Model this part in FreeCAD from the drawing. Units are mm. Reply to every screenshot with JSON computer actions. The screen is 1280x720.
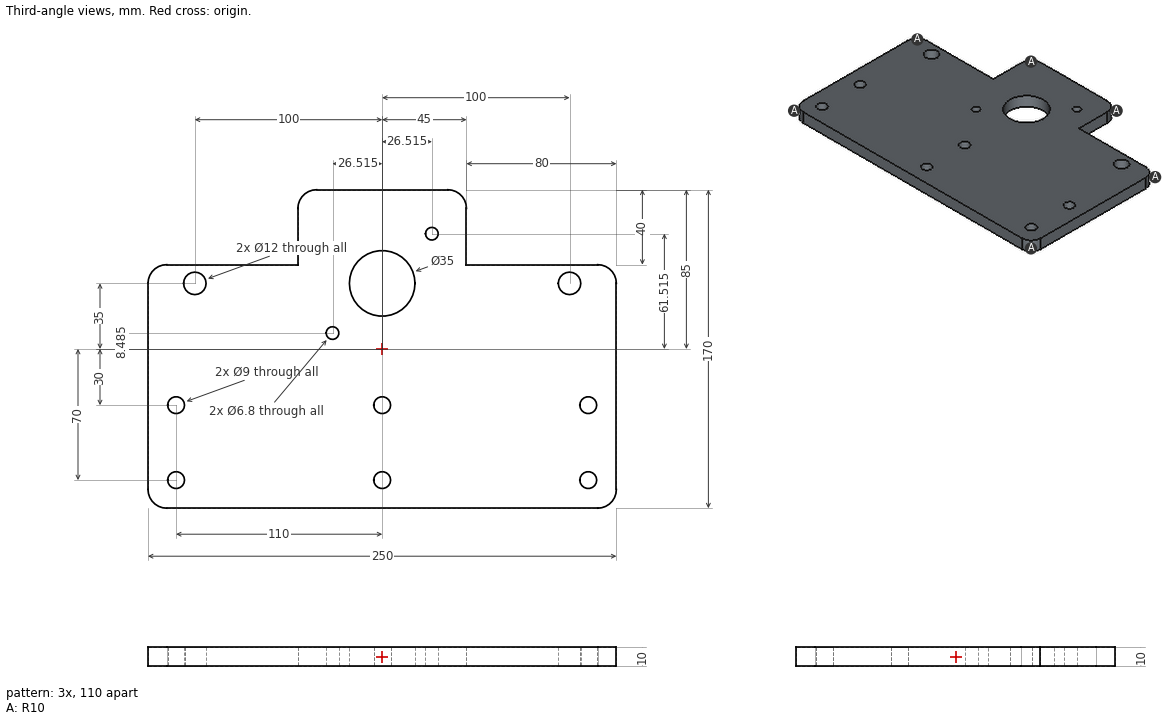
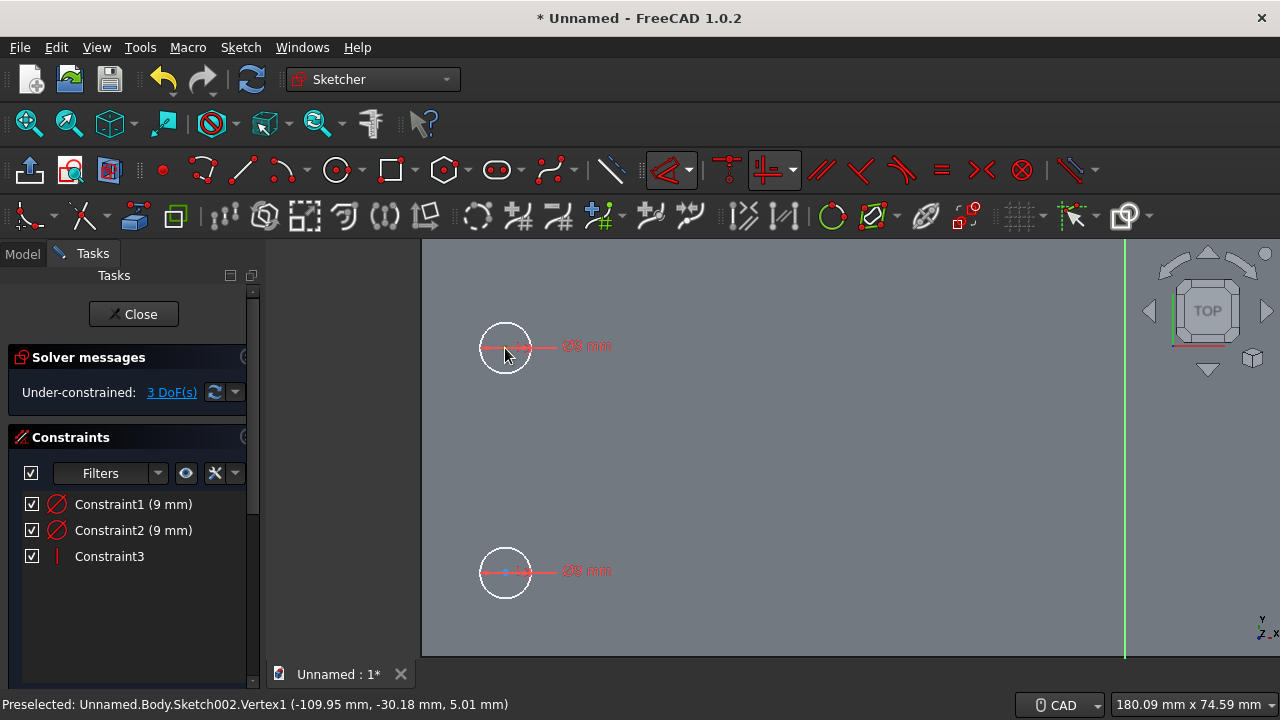
{"action": "left_click", "coordinate": [692, 170]}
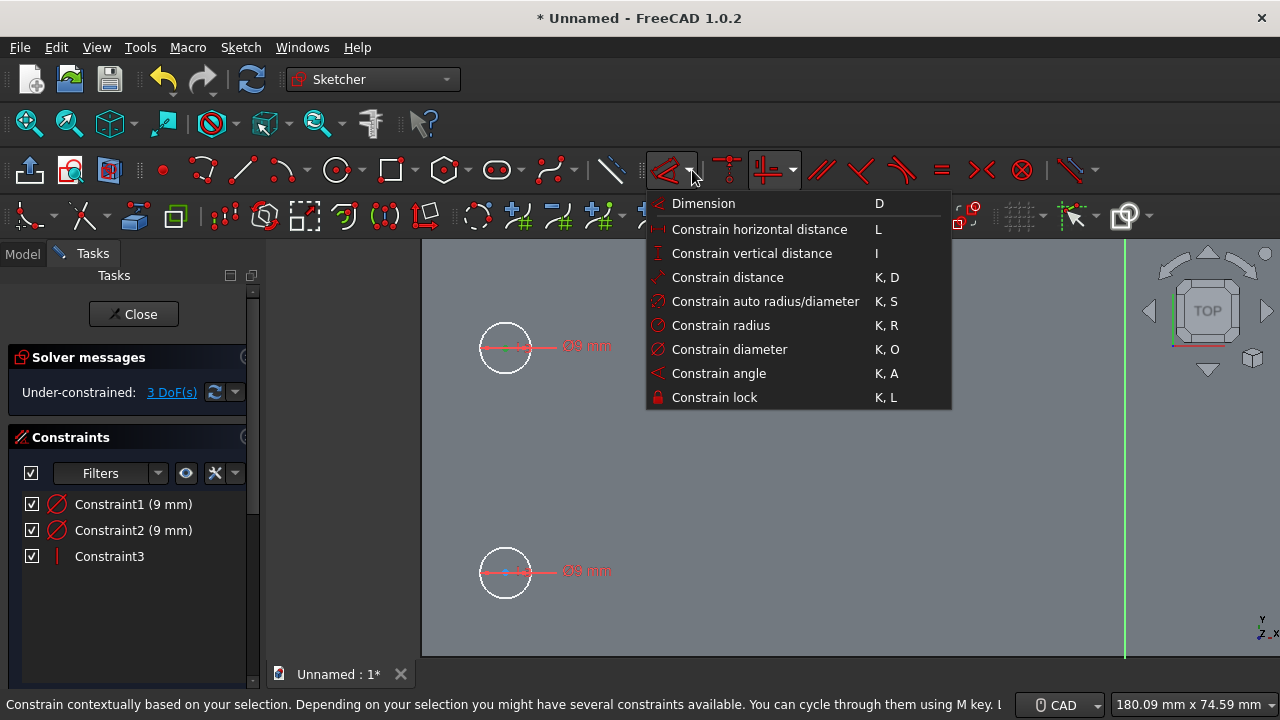
{"action": "left_click", "coordinate": [799, 253]}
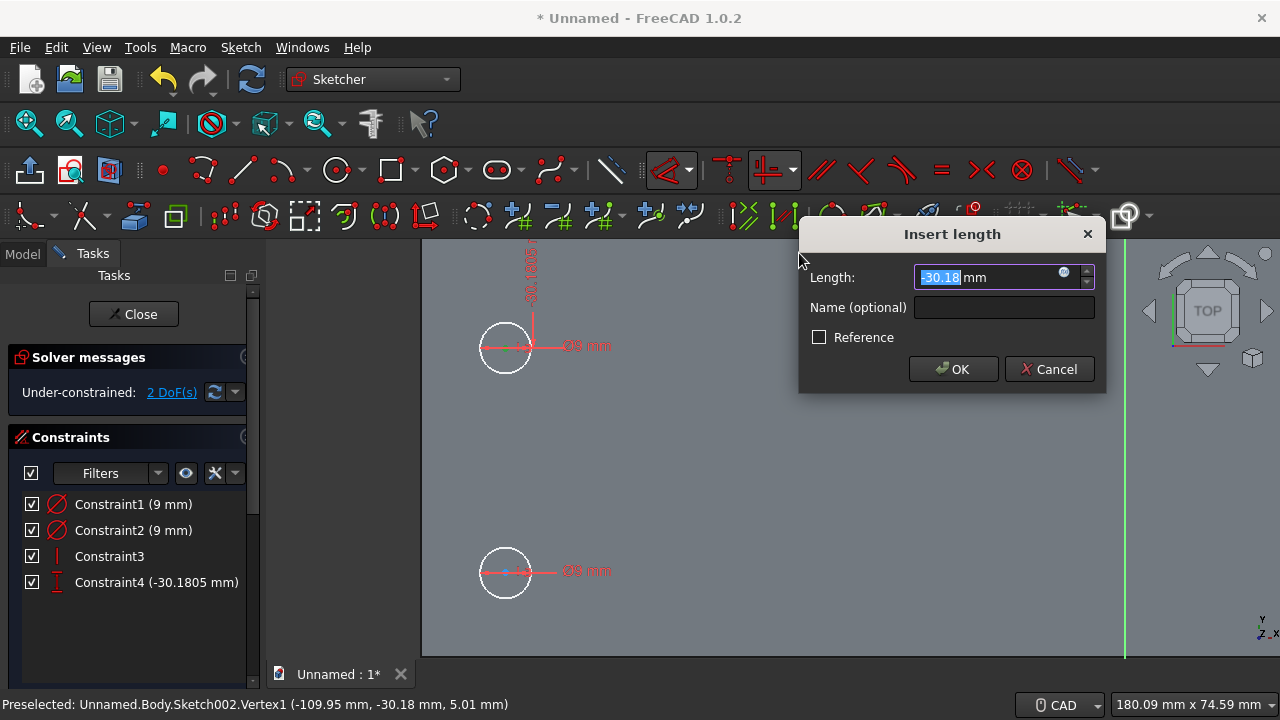
{"action": "type", "text": "-30"}
{"action": "key", "text": "Return"}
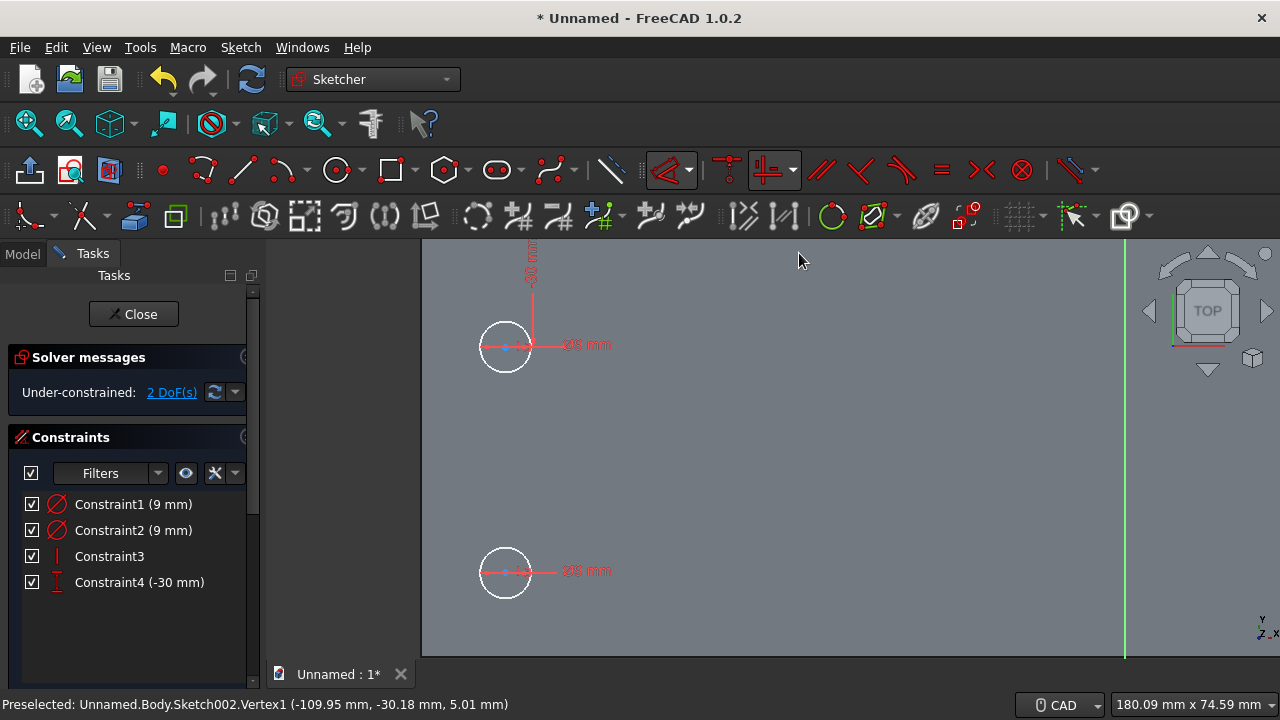
{"action": "left_click", "coordinate": [505, 573]}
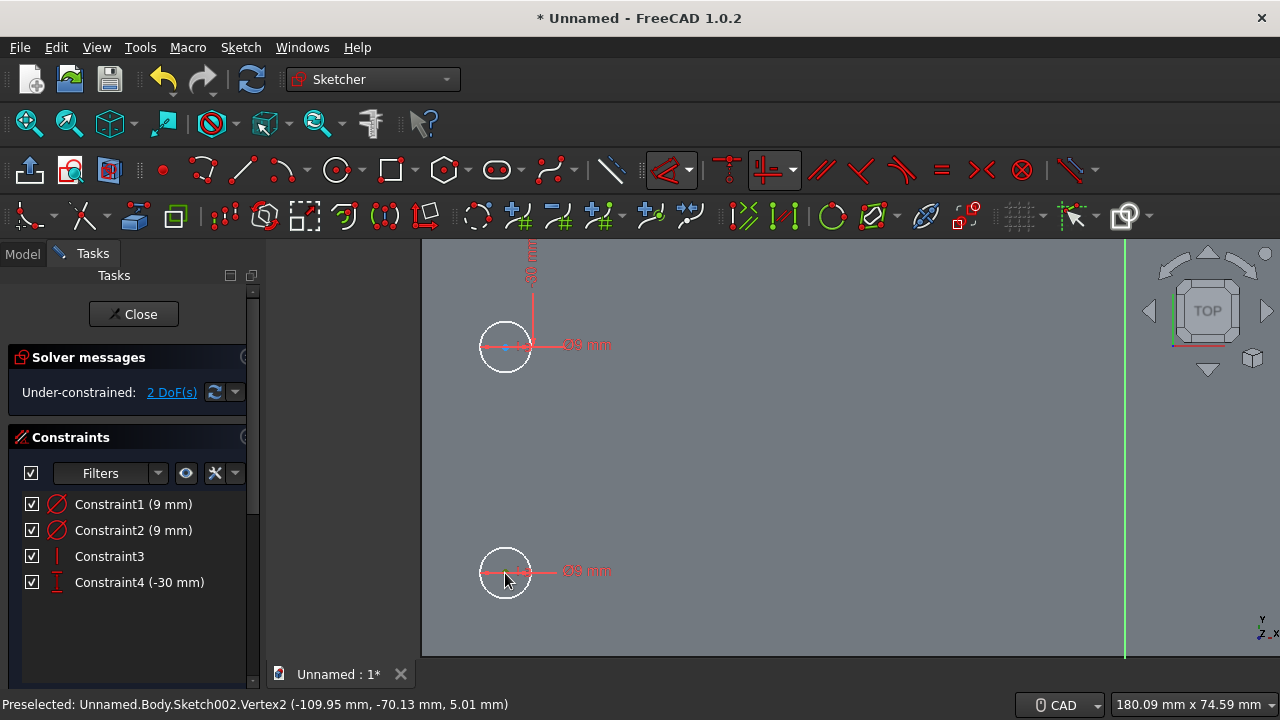
{"action": "key", "text": "i"}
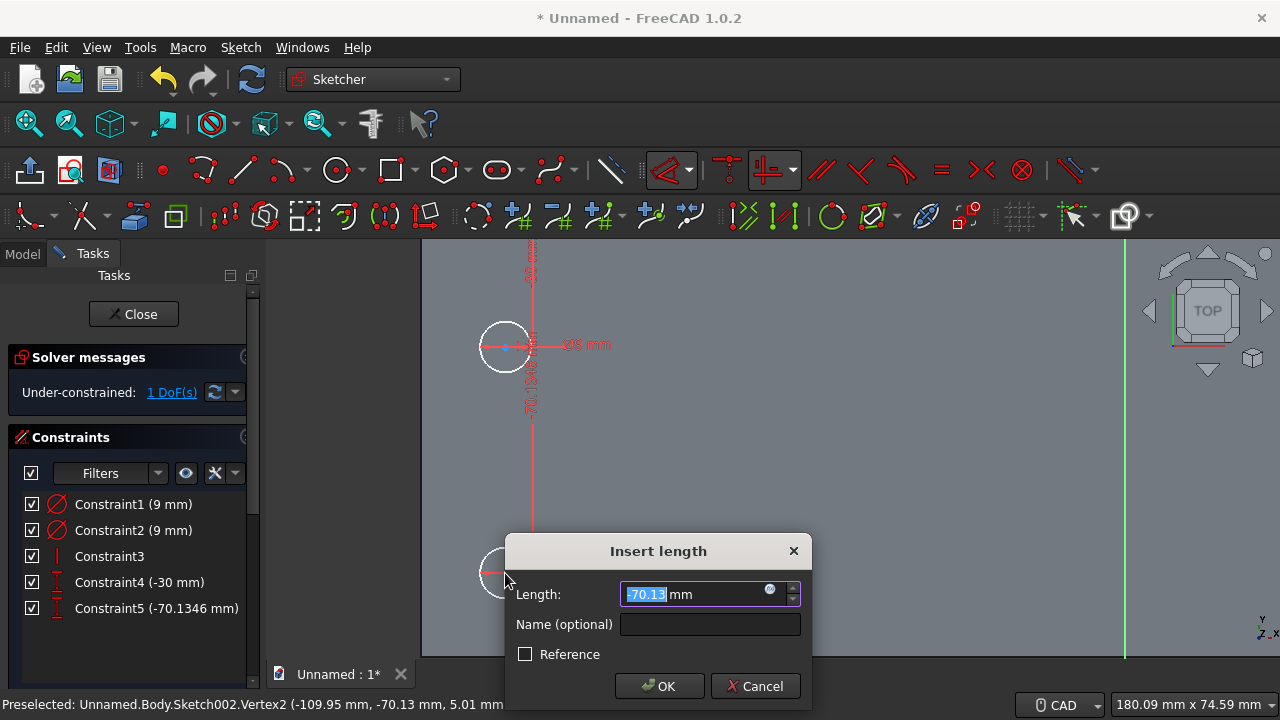
{"action": "type", "text": "-70"}
{"action": "key", "text": "Return"}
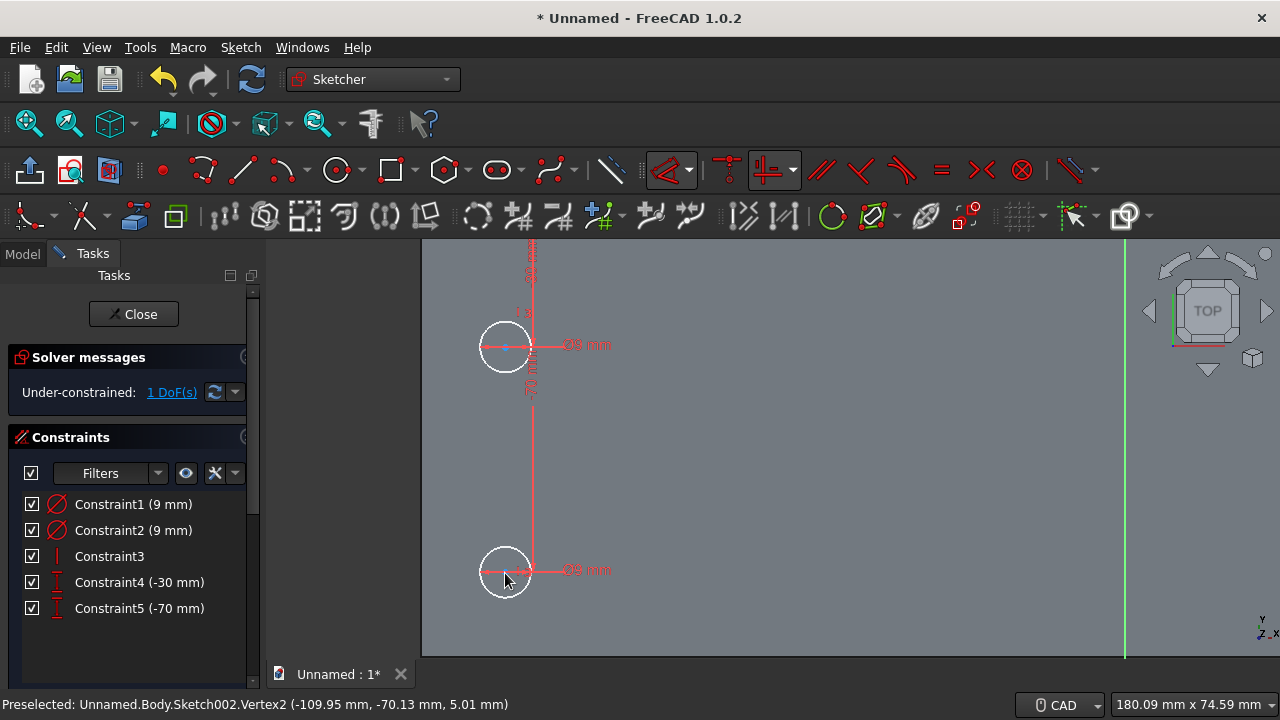
{"action": "left_click", "coordinate": [505, 347]}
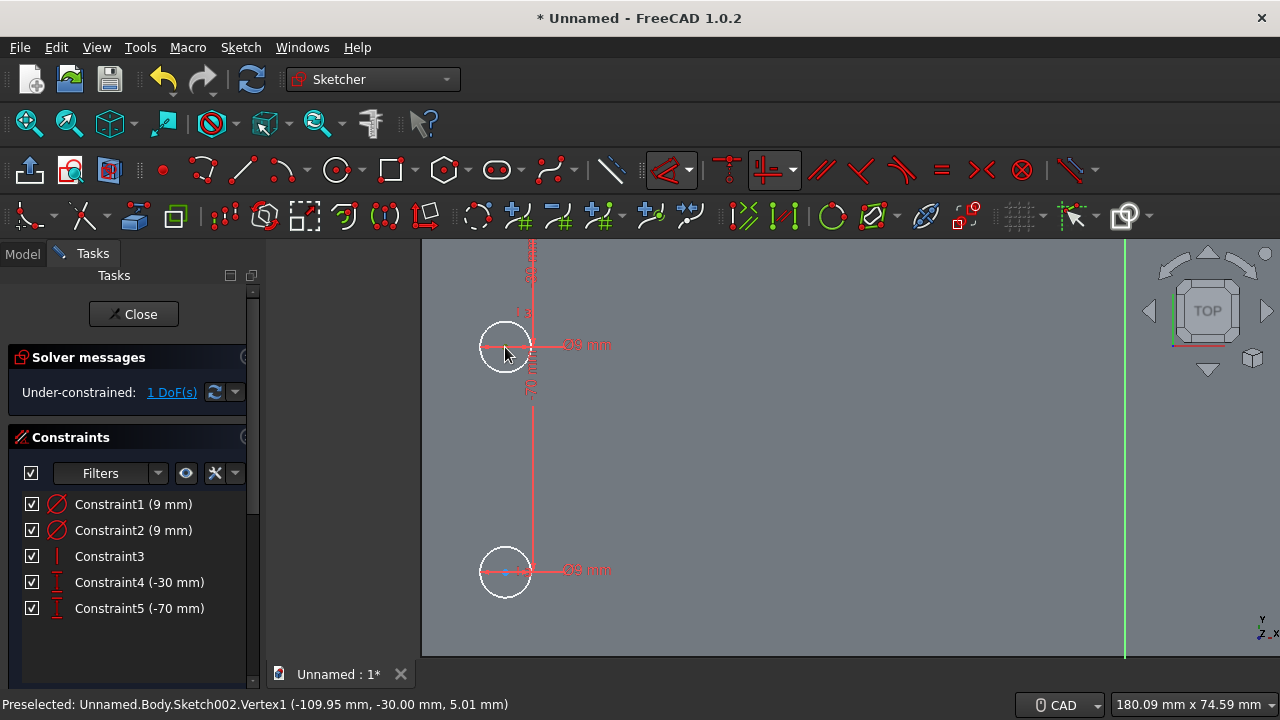
{"action": "left_click", "coordinate": [692, 170]}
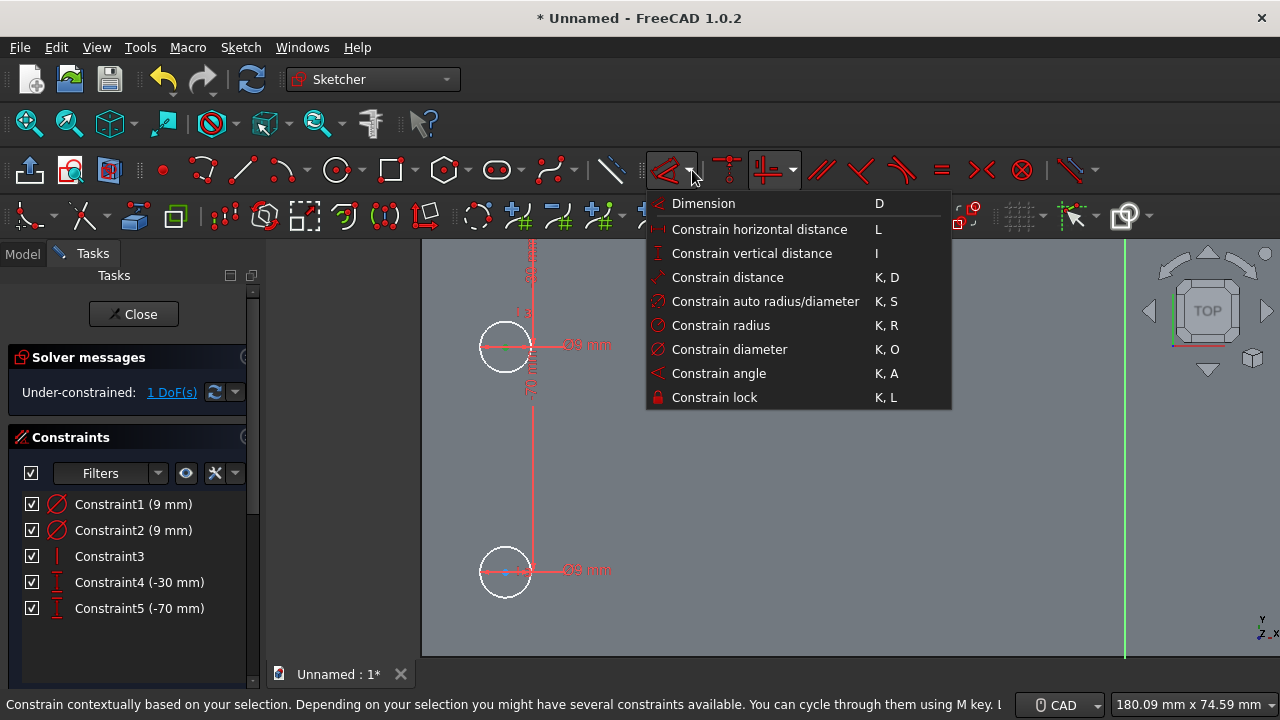
{"action": "left_click", "coordinate": [799, 229]}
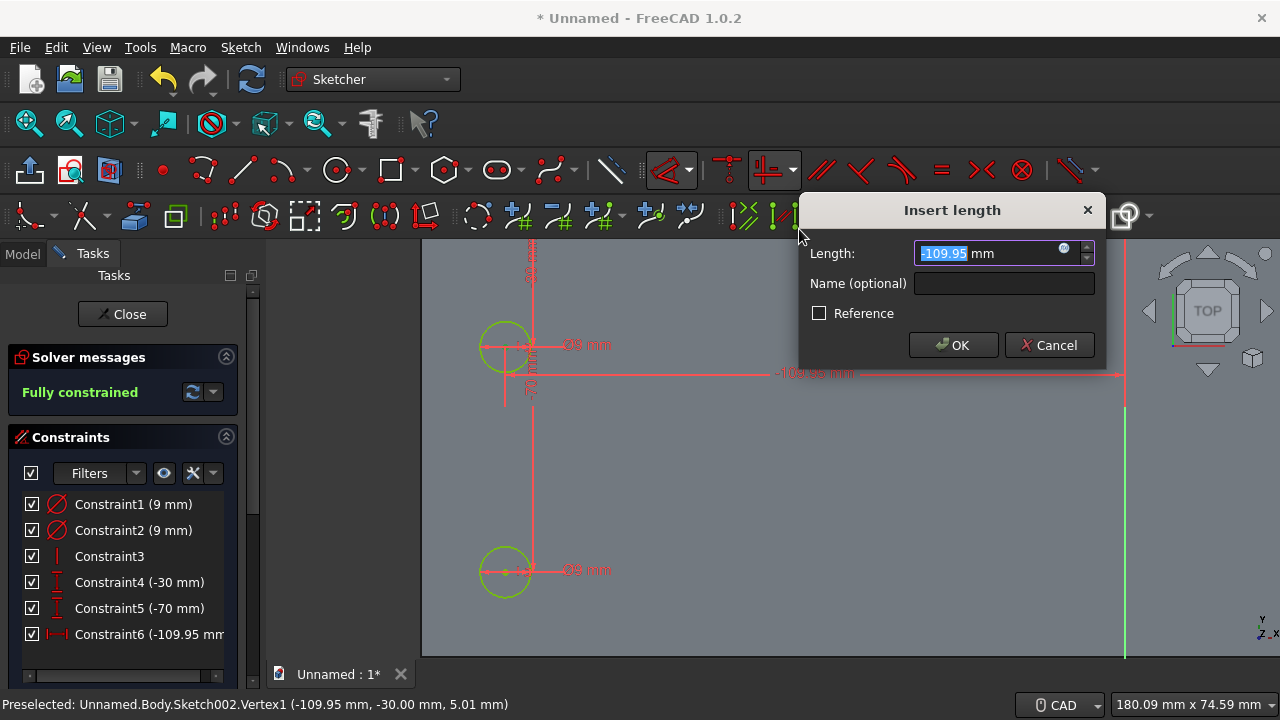
{"action": "type", "text": "-110"}
{"action": "key", "text": "Return"}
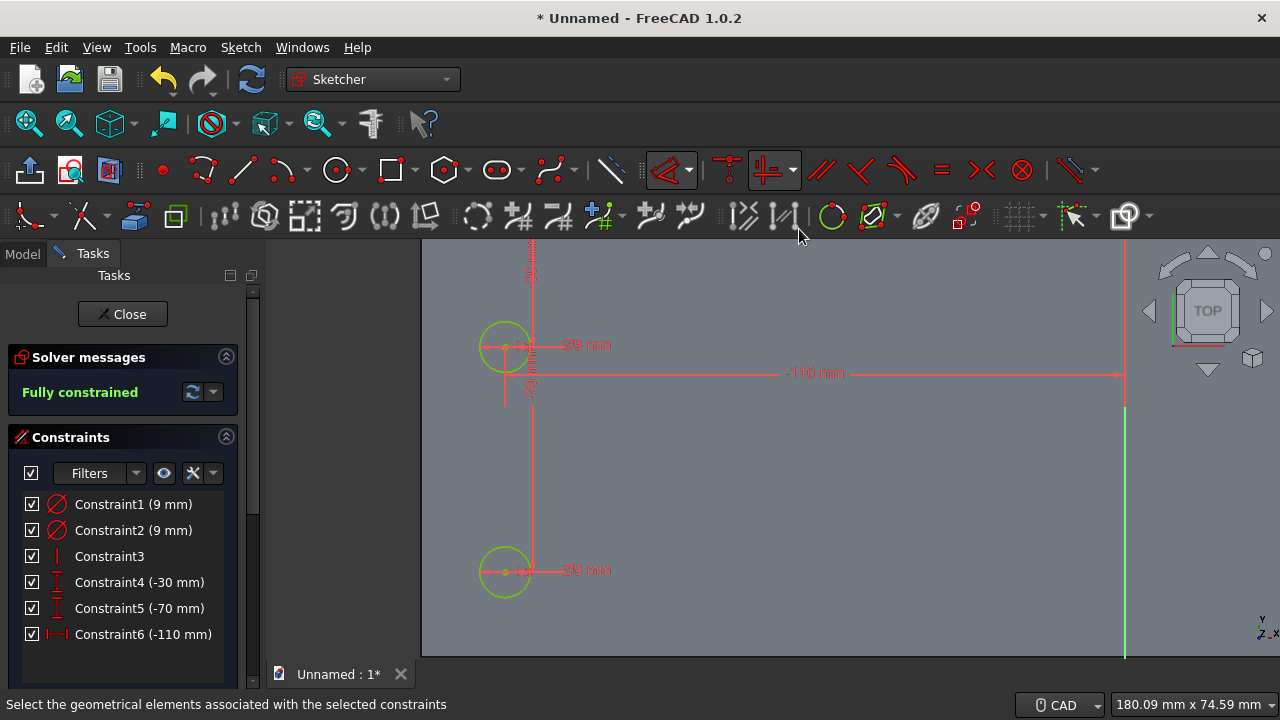
{"action": "left_click", "coordinate": [123, 314]}